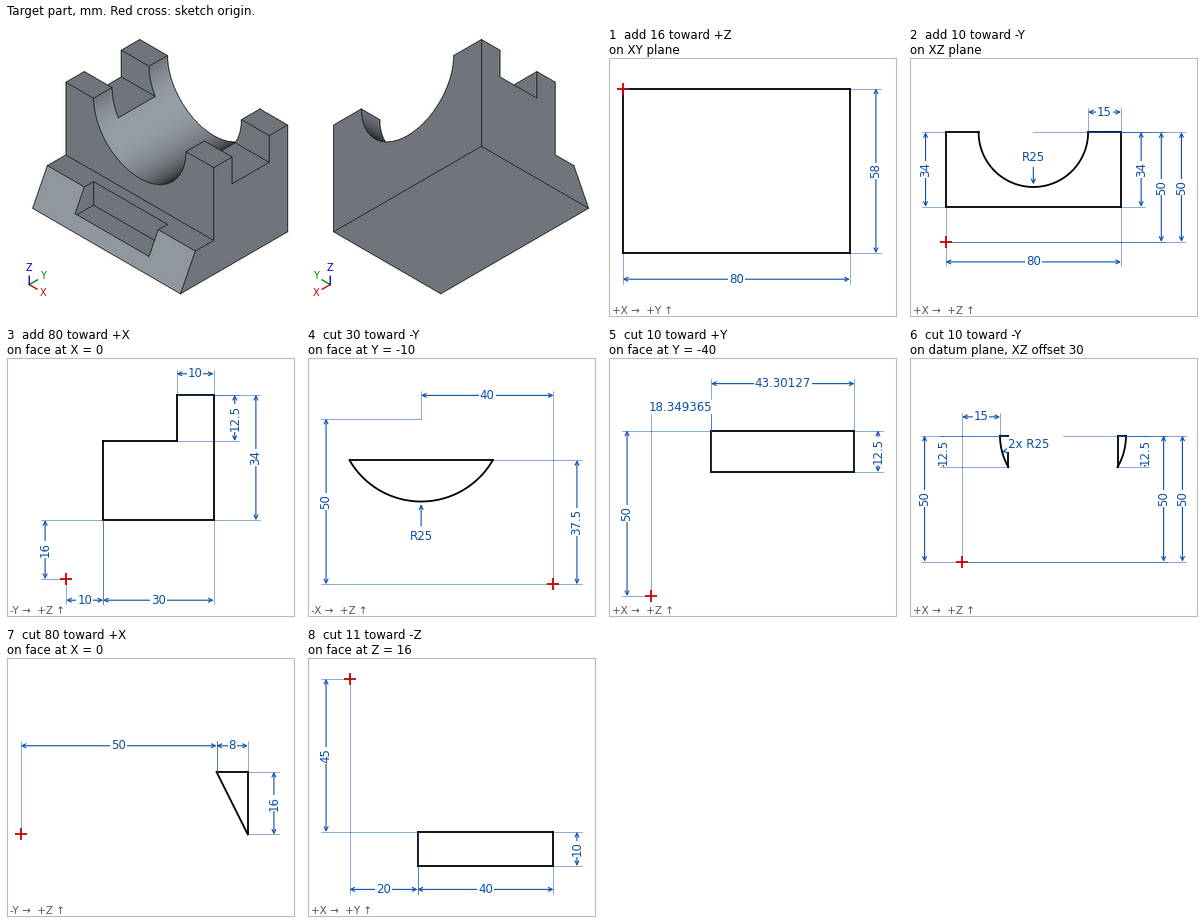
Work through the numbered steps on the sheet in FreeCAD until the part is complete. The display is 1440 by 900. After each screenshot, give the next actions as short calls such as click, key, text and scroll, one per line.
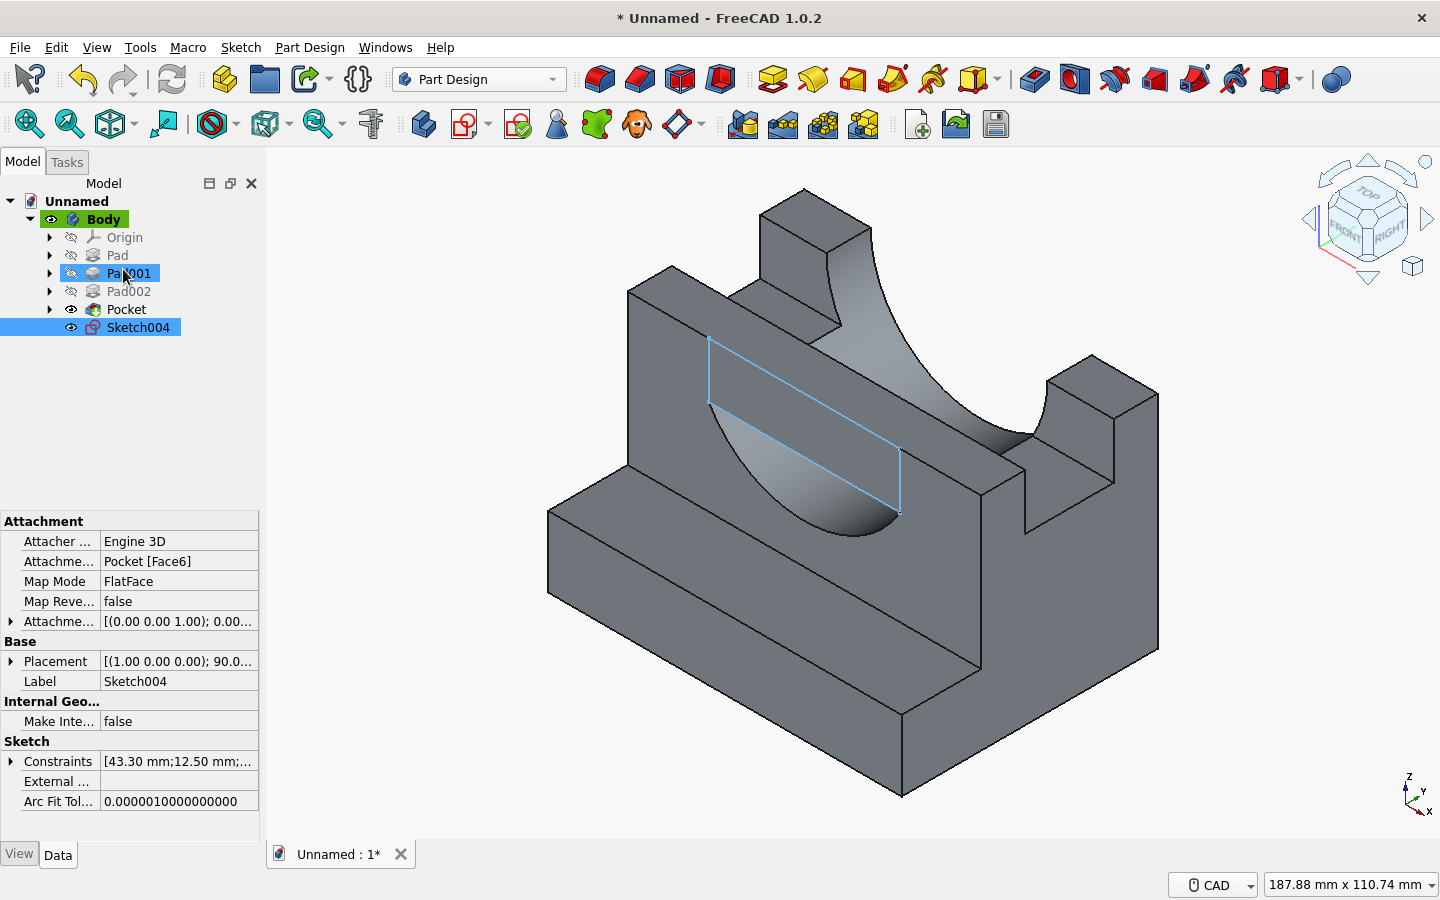
click(1036, 80)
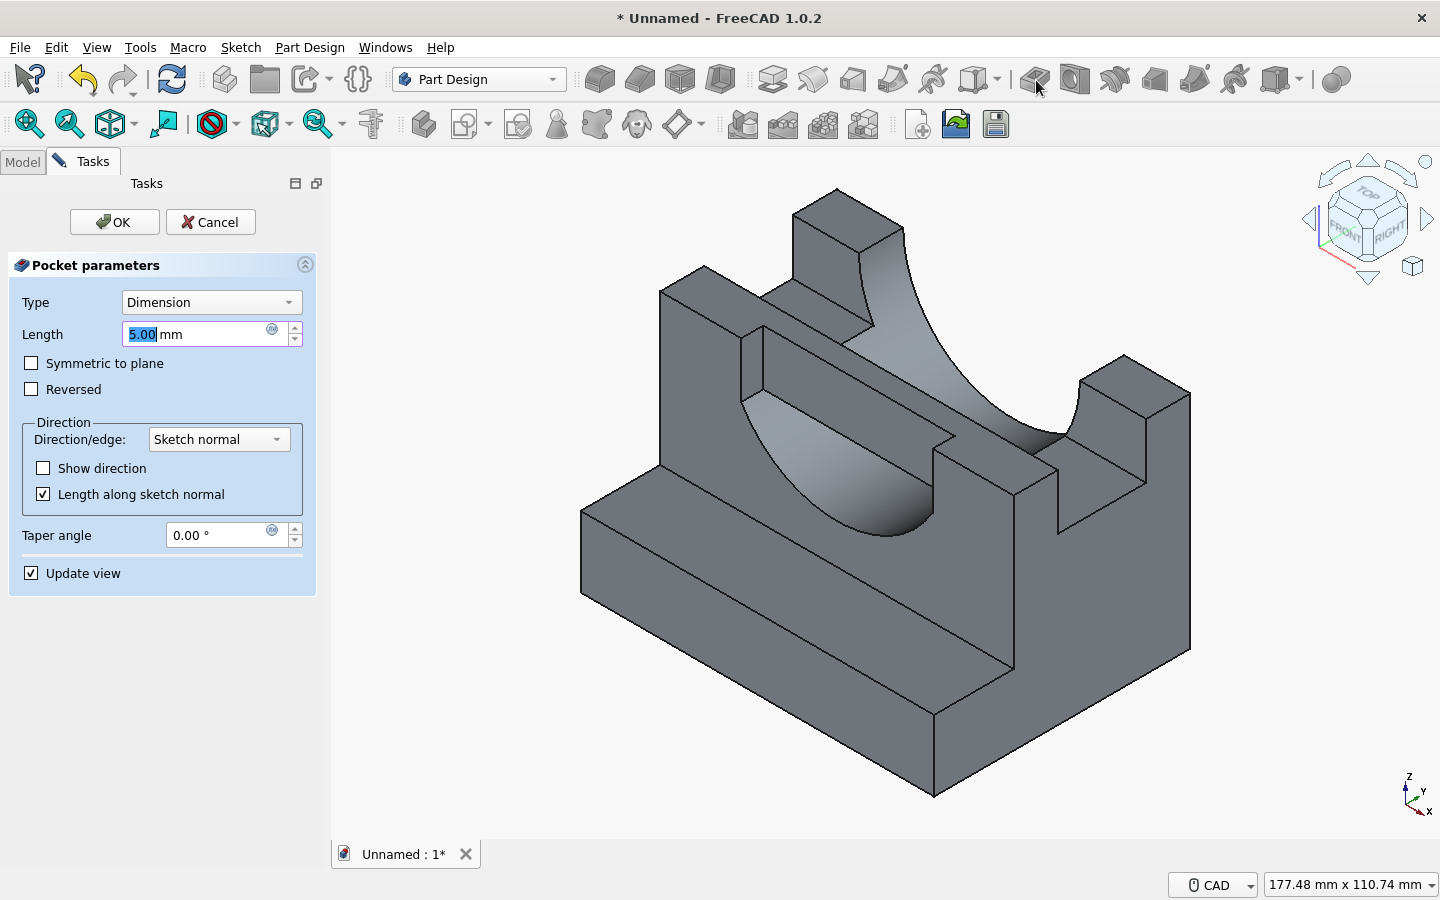
text(10)
key(Tab)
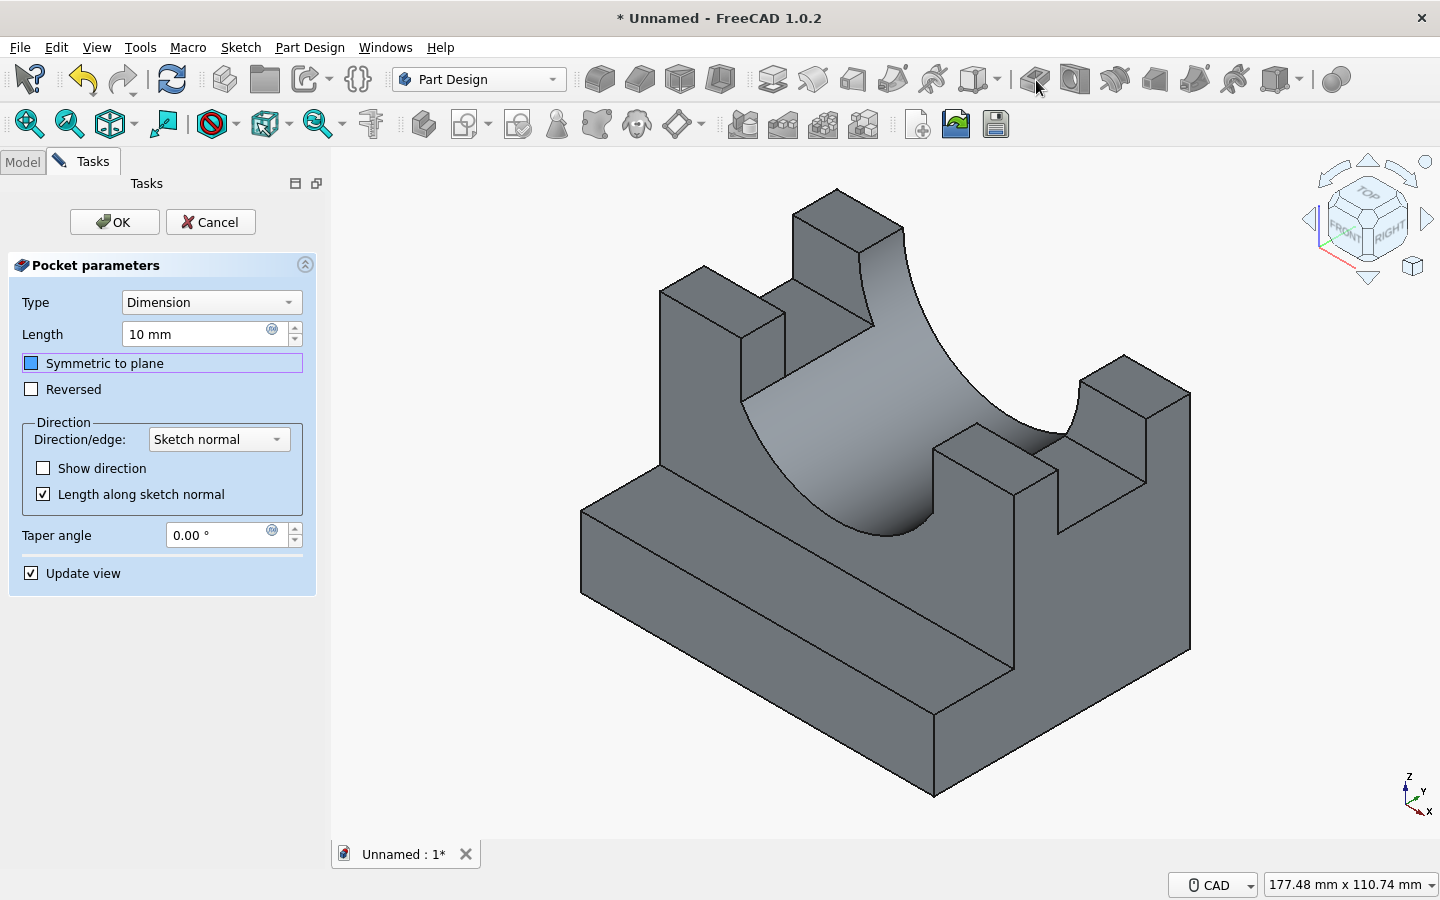
click(115, 222)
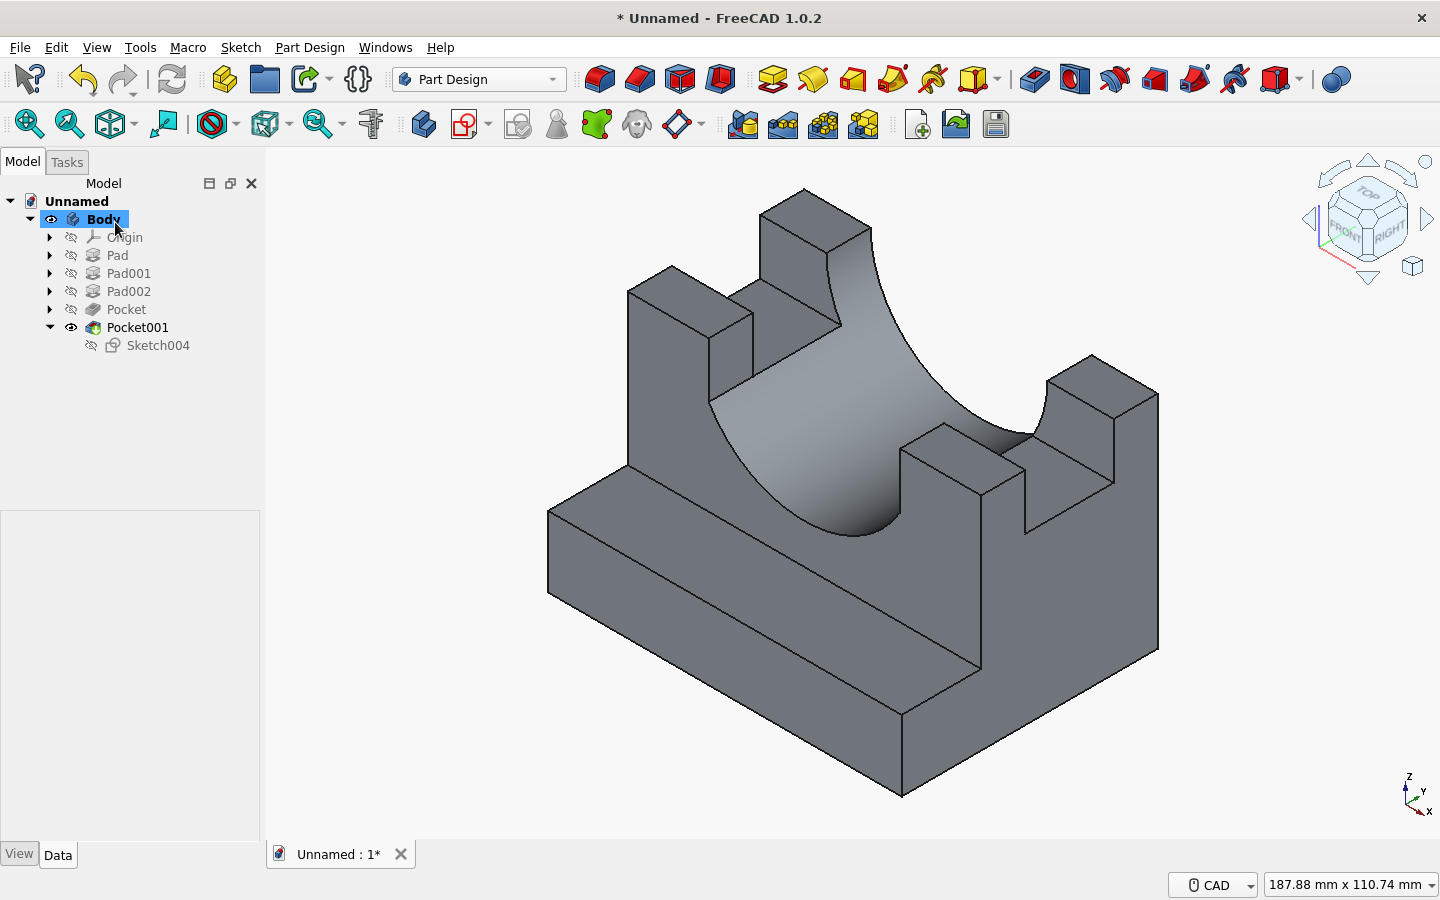
click(50, 237)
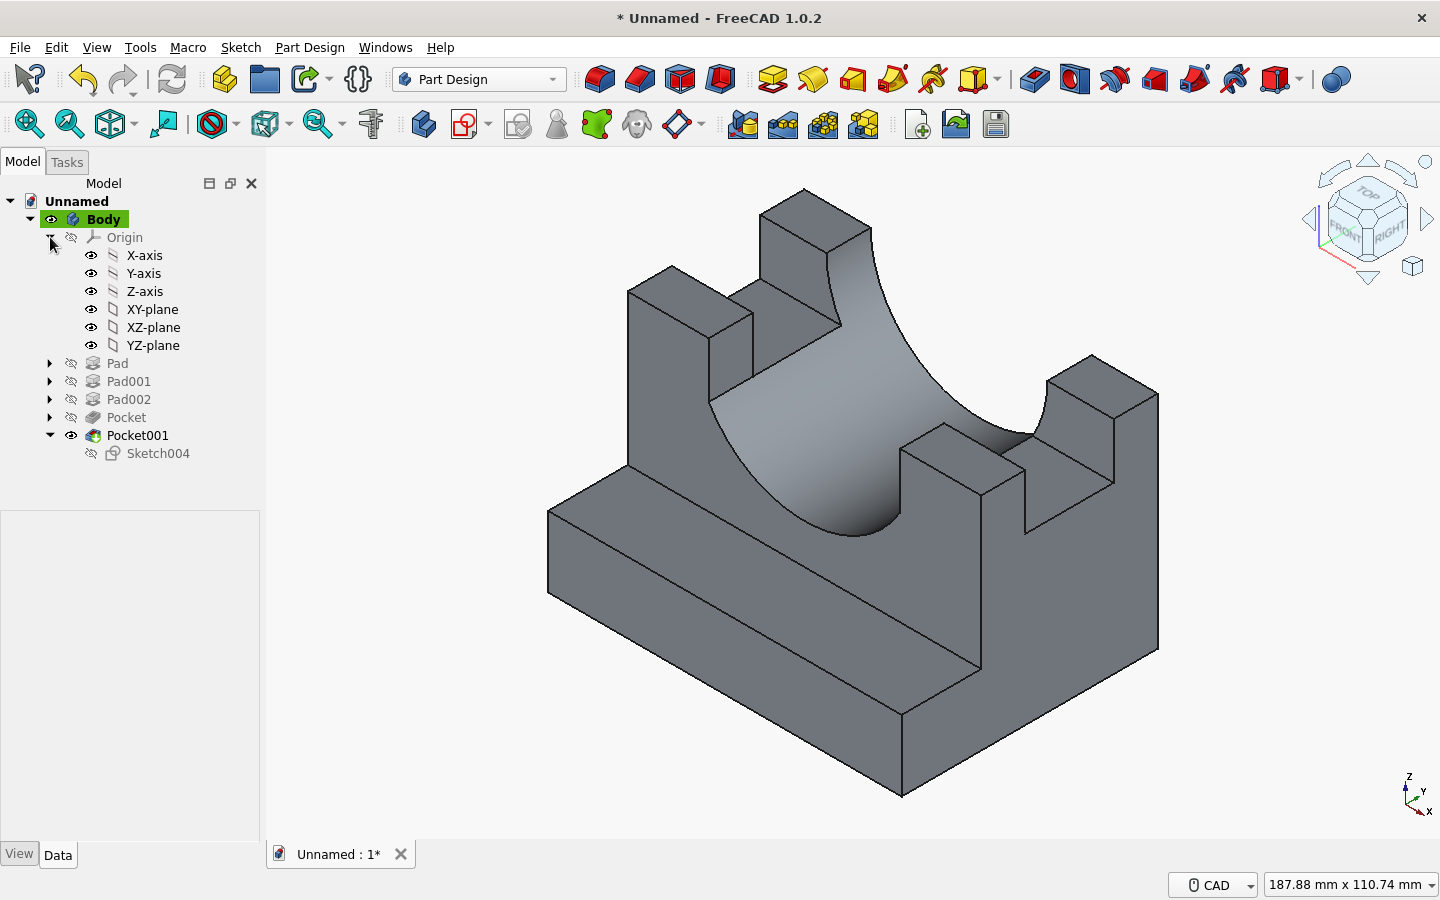
click(136, 327)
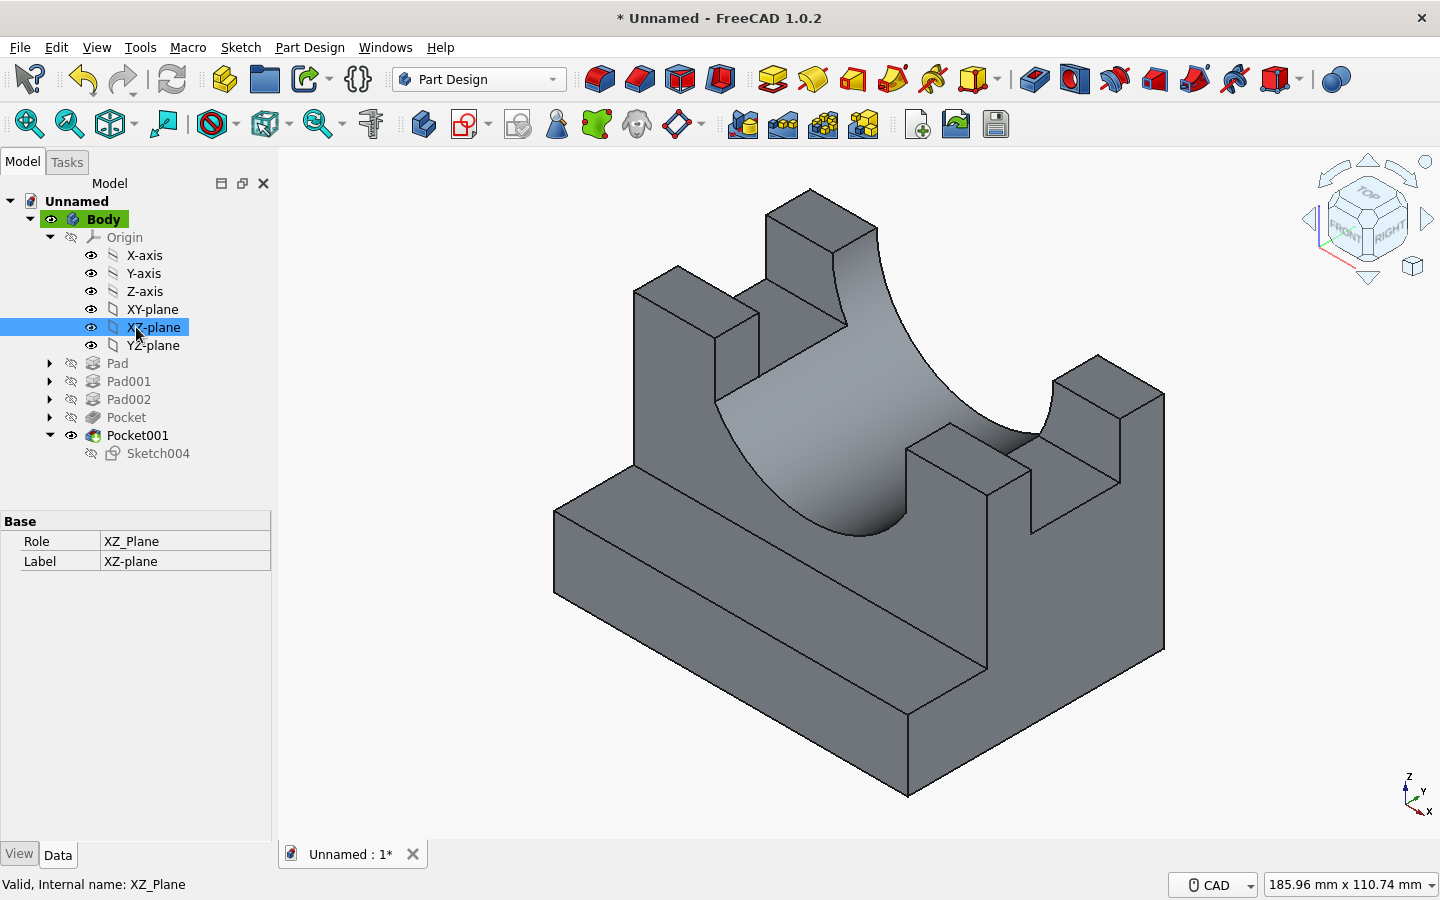
click(678, 124)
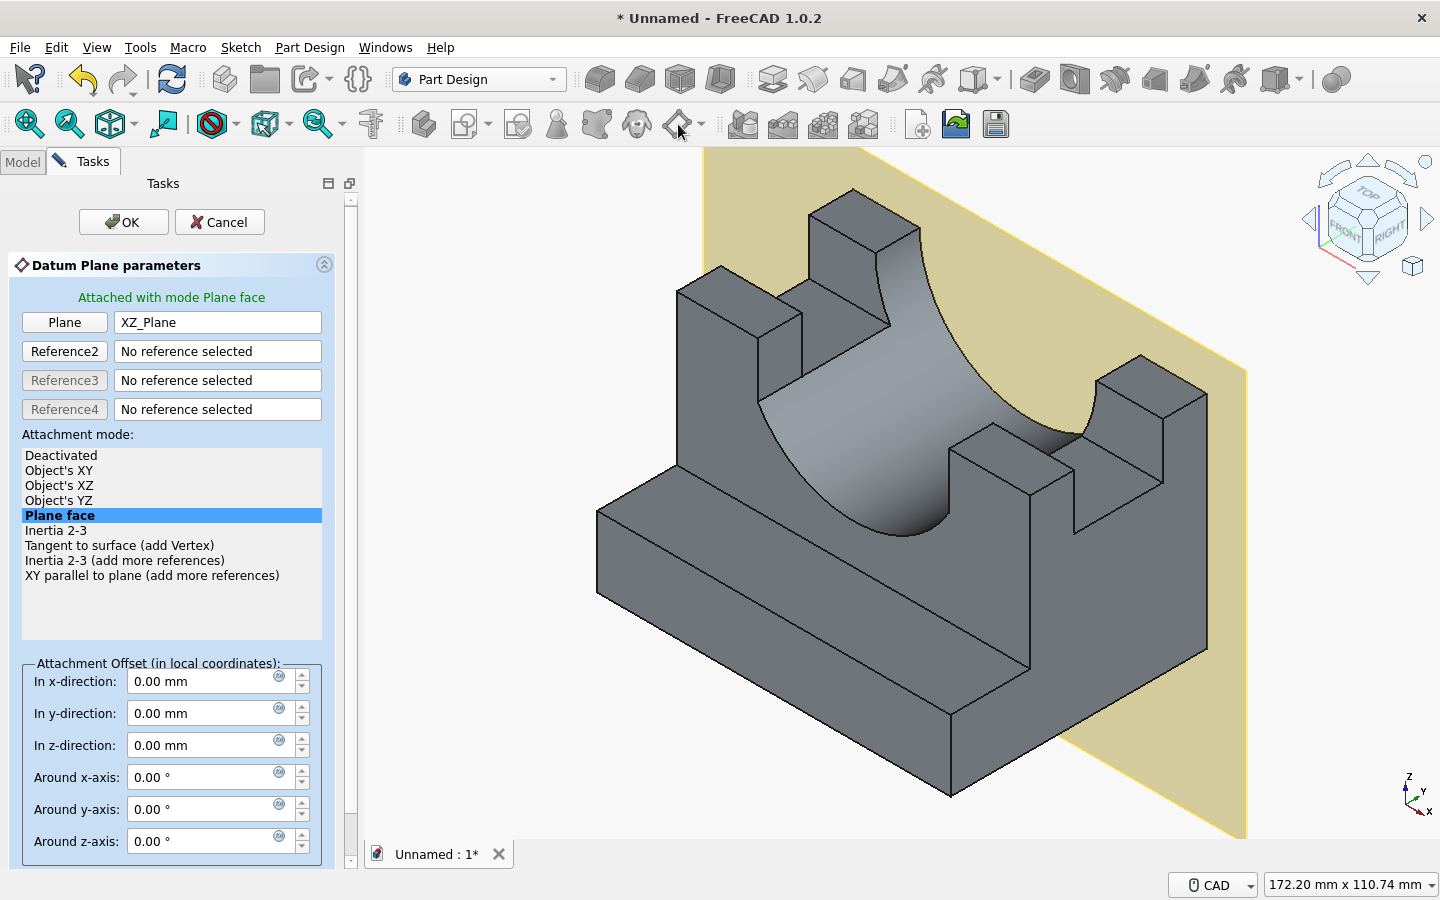
triple_click(210, 745)